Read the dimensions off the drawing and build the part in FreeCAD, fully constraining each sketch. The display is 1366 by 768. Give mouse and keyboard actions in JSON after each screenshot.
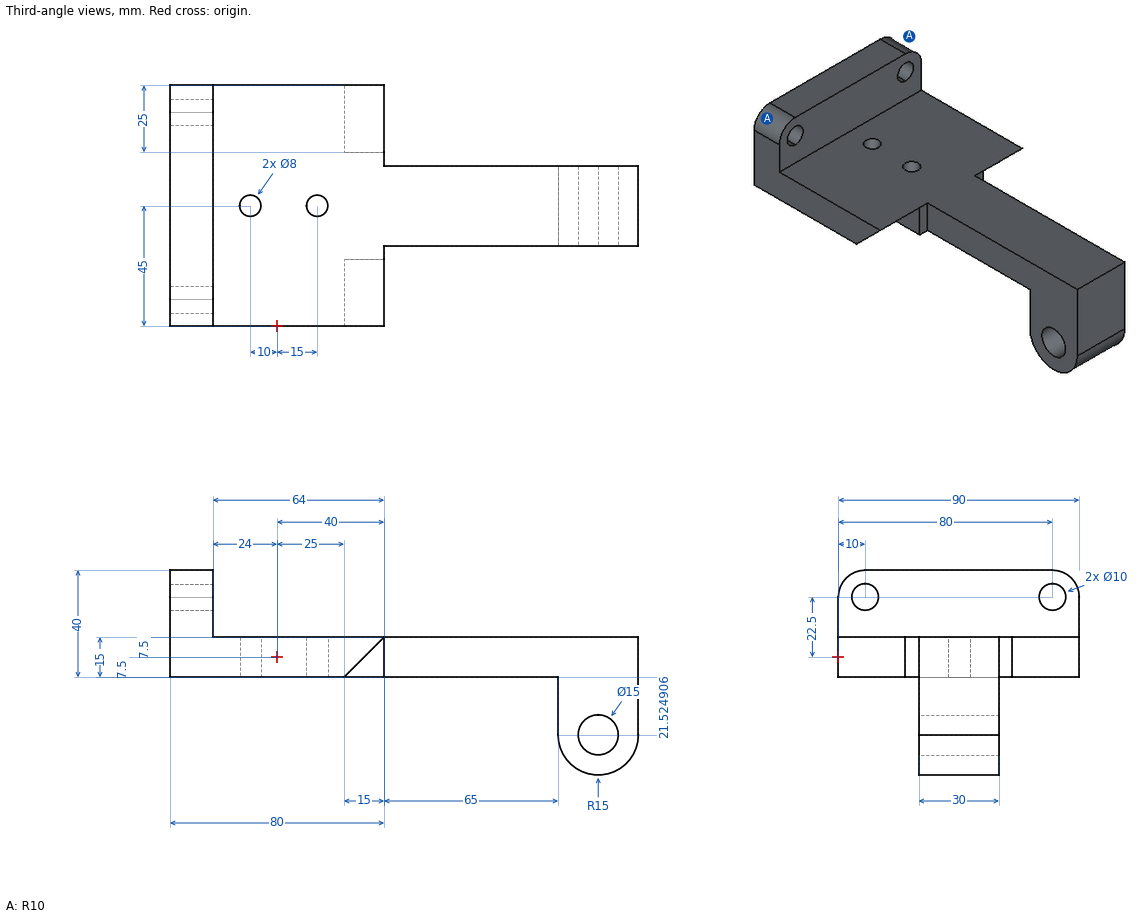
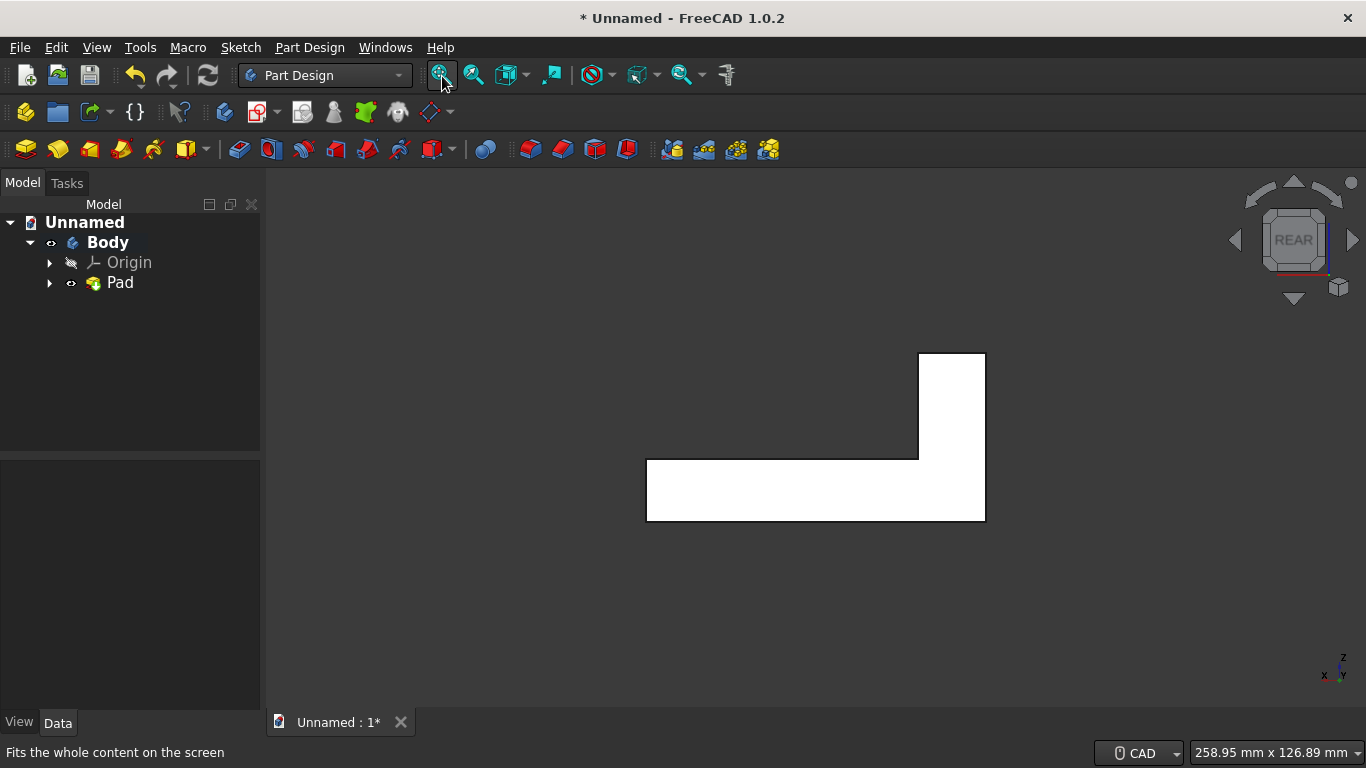
{"action": "left_click", "coordinate": [442, 76]}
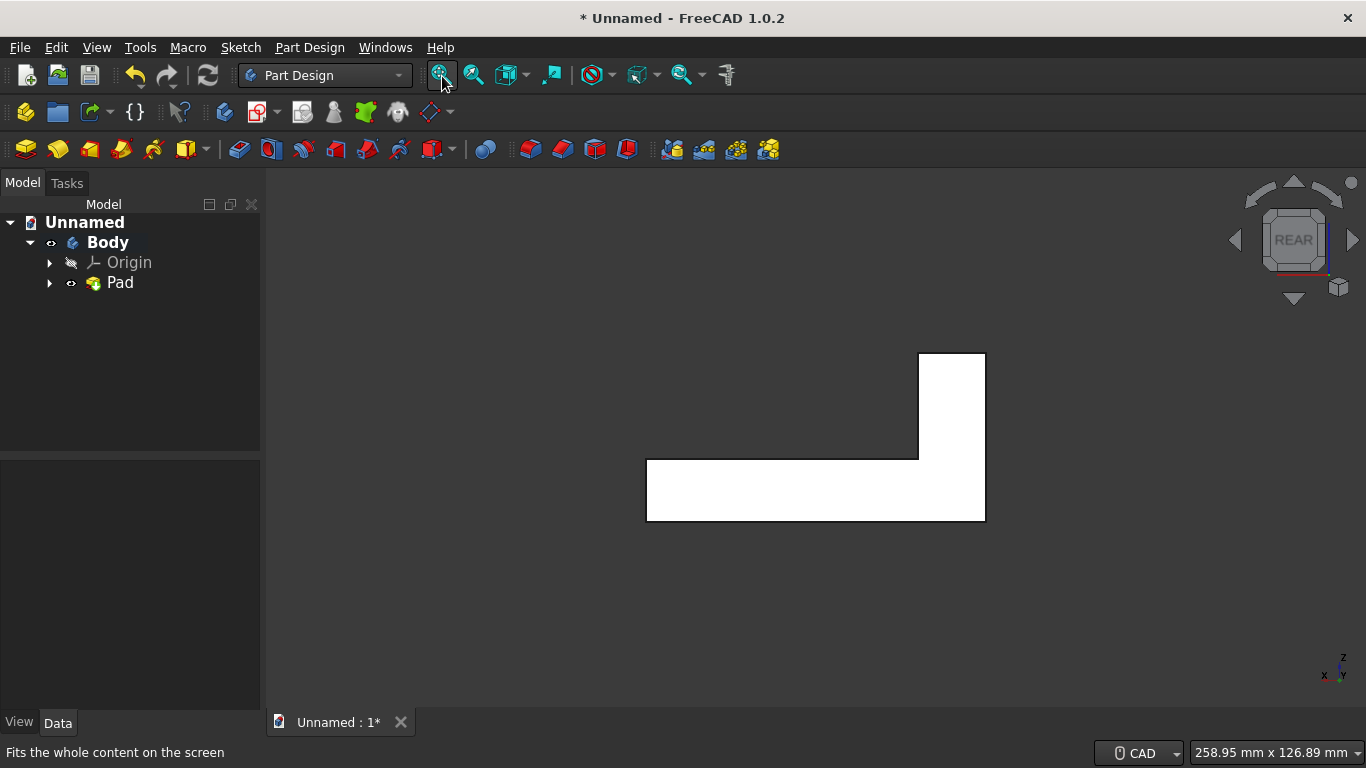
{"action": "left_click", "coordinate": [719, 485]}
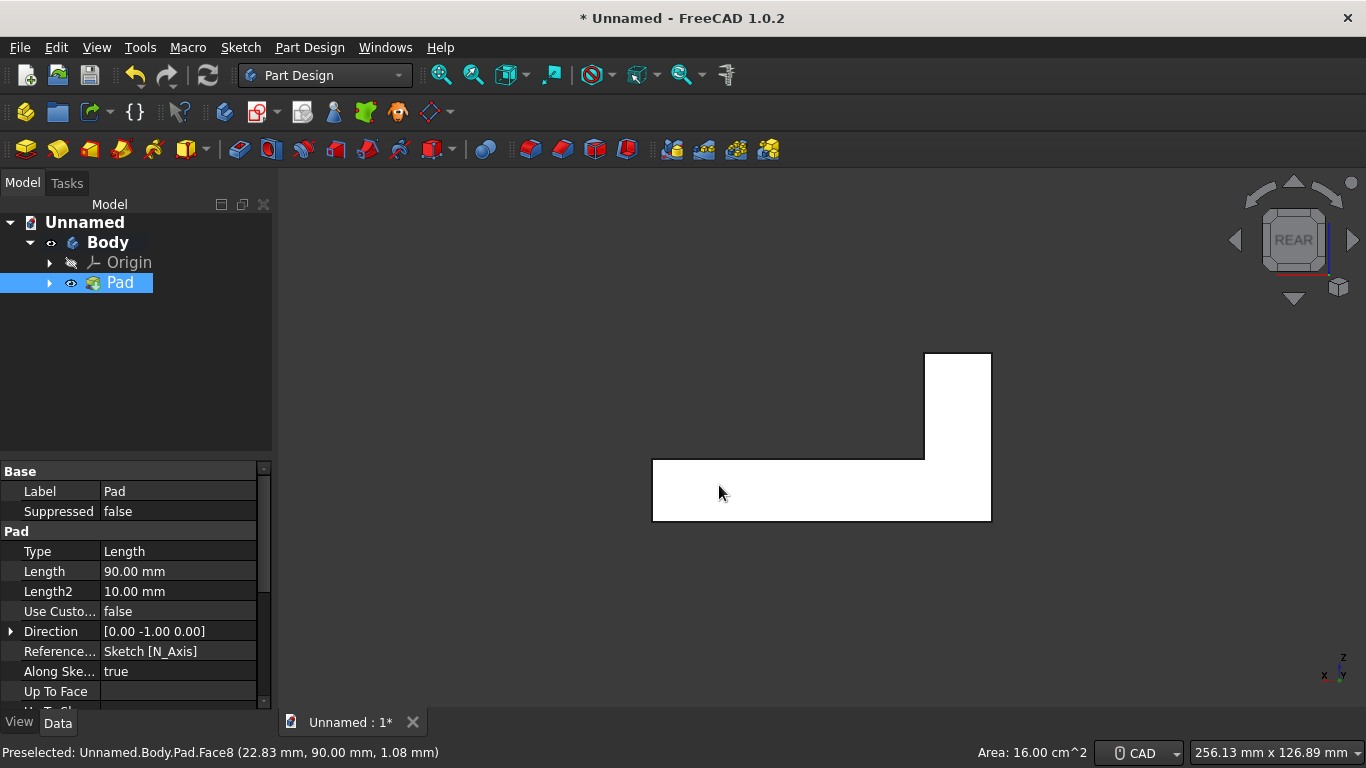
{"action": "left_click", "coordinate": [258, 112]}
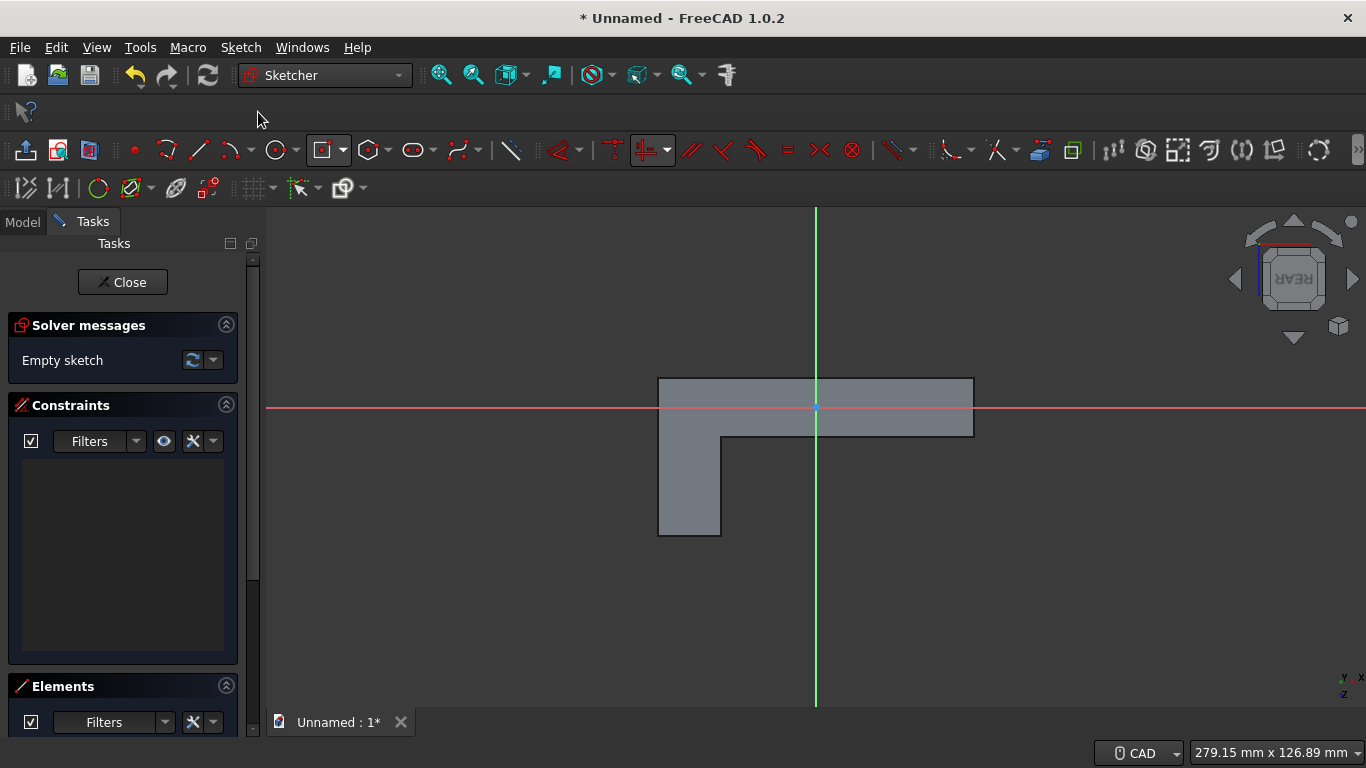
{"action": "scroll", "coordinate": [994, 395], "scroll_direction": "up", "scroll_amount": 8}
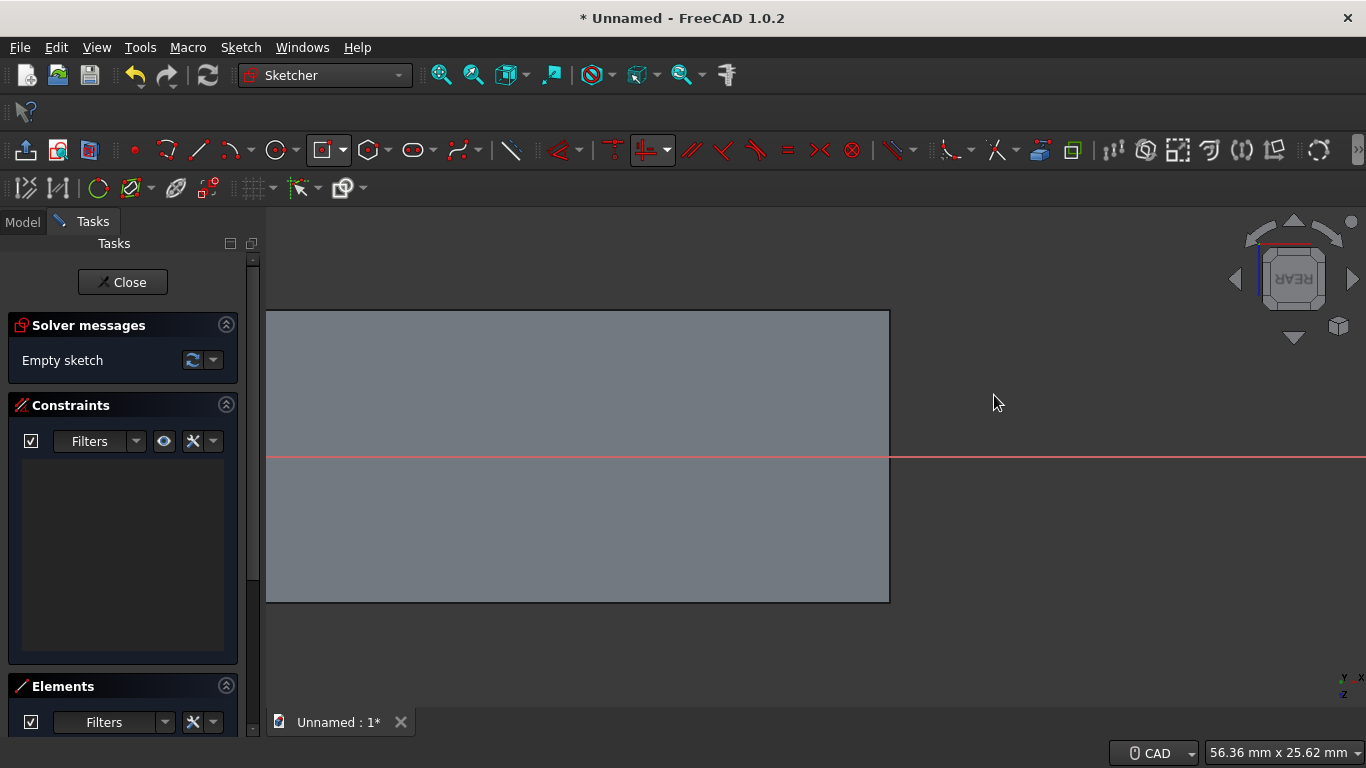
{"action": "left_click", "coordinate": [168, 150]}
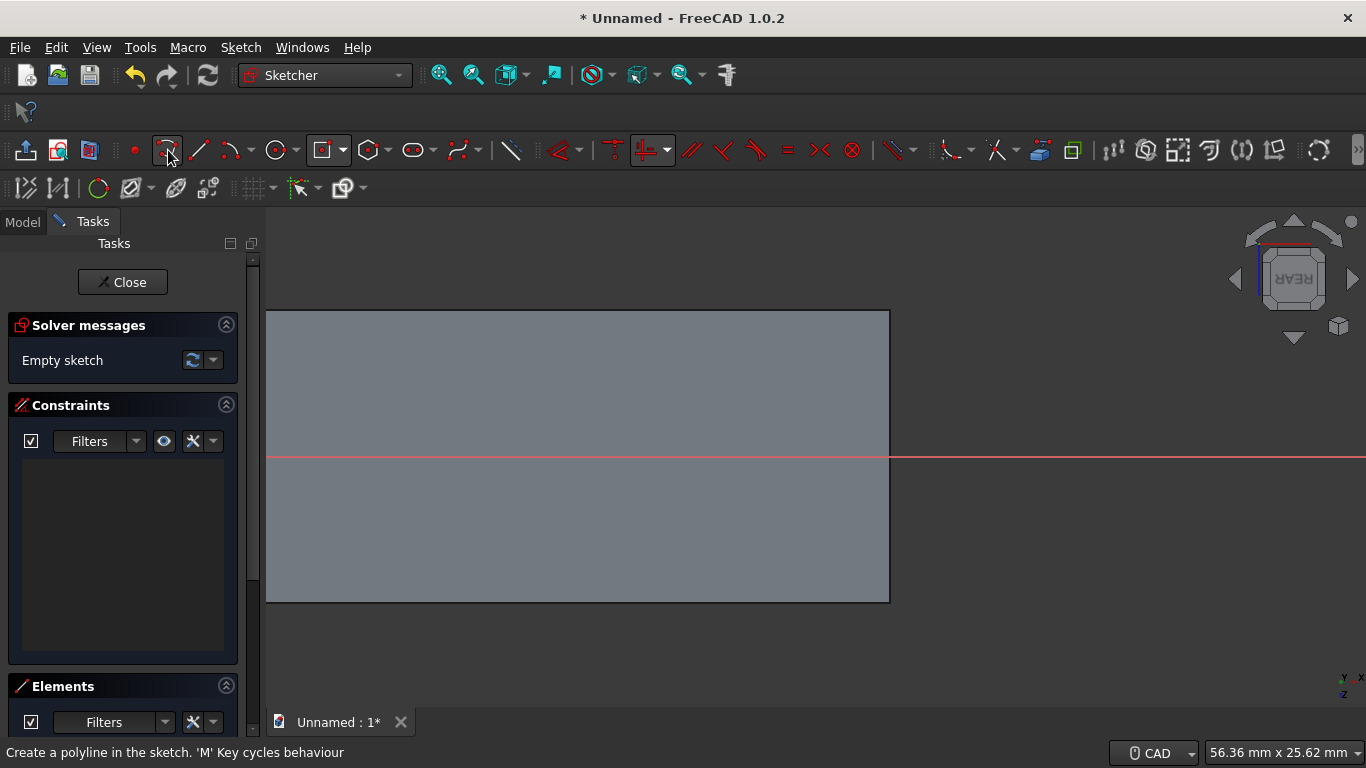
{"action": "left_click", "coordinate": [598, 310]}
{"action": "left_click", "coordinate": [890, 603]}
{"action": "left_click", "coordinate": [890, 310]}
{"action": "left_click", "coordinate": [598, 311]}
{"action": "key", "text": "Escape"}
{"action": "key", "text": "Escape"}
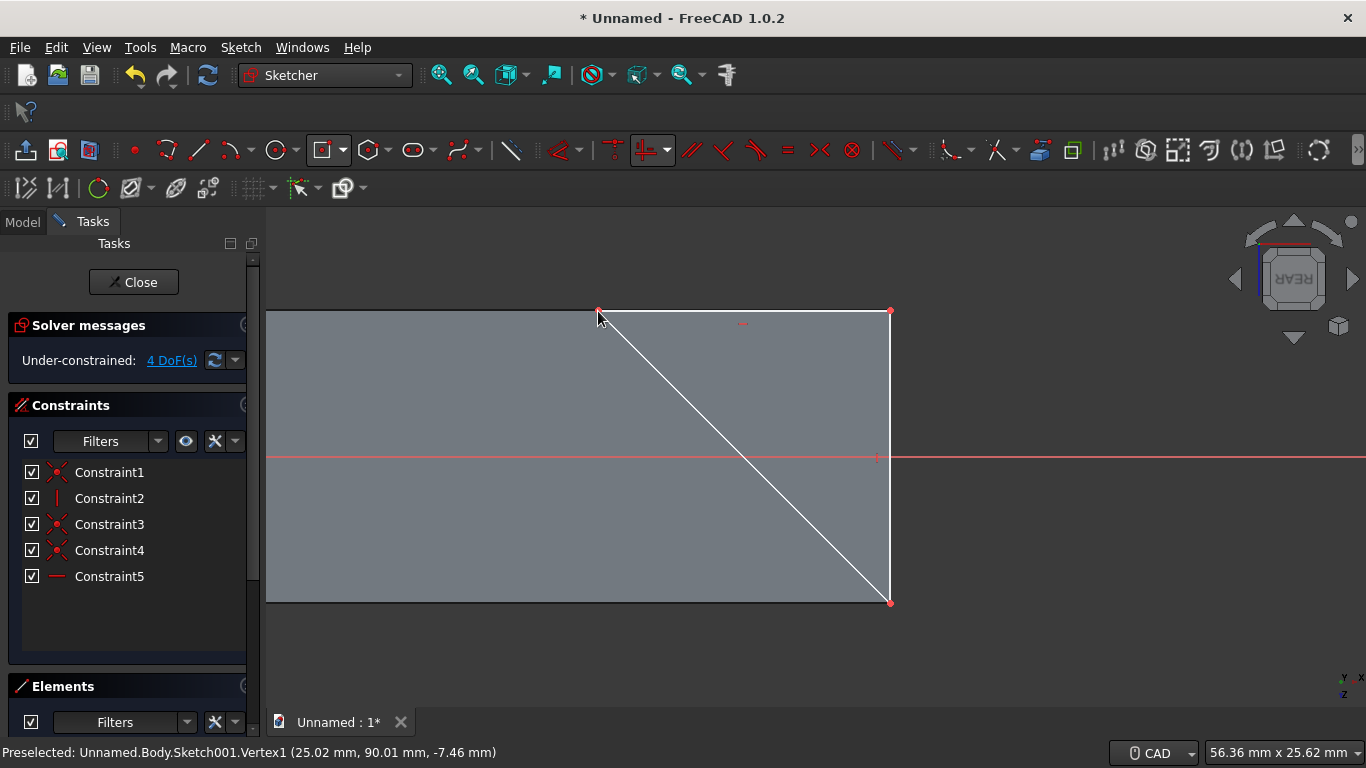
{"action": "left_click", "coordinate": [558, 150]}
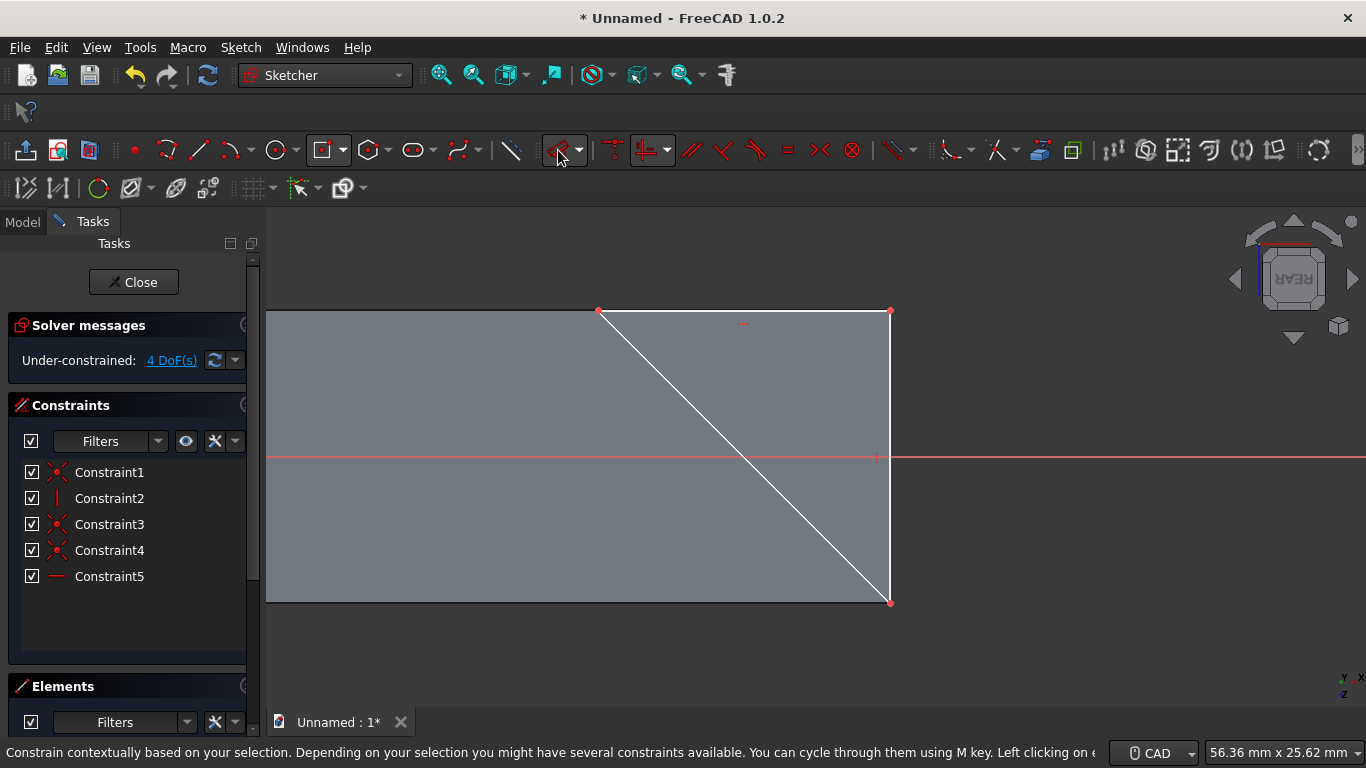
{"action": "left_click", "coordinate": [890, 516]}
{"action": "left_click", "coordinate": [924, 390]}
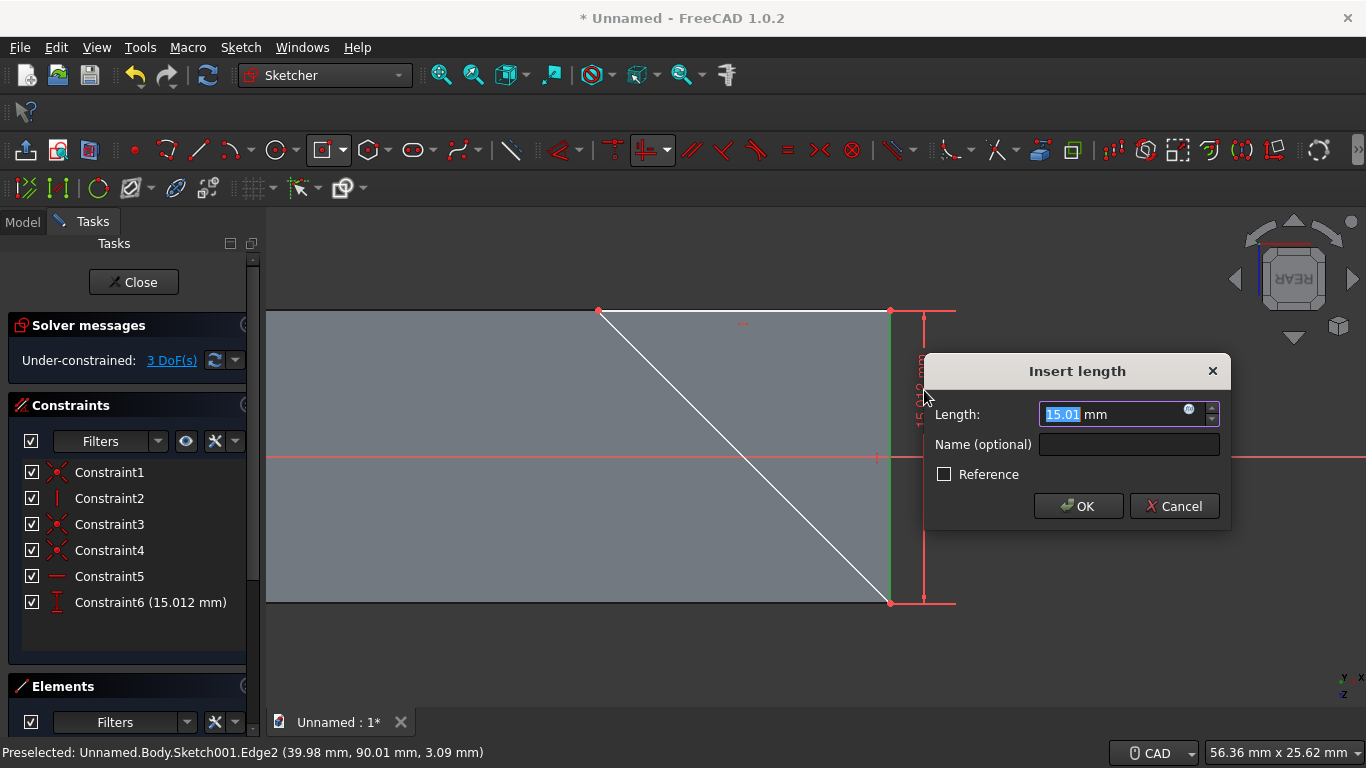
{"action": "type", "text": "15"}
{"action": "key", "text": "Return"}